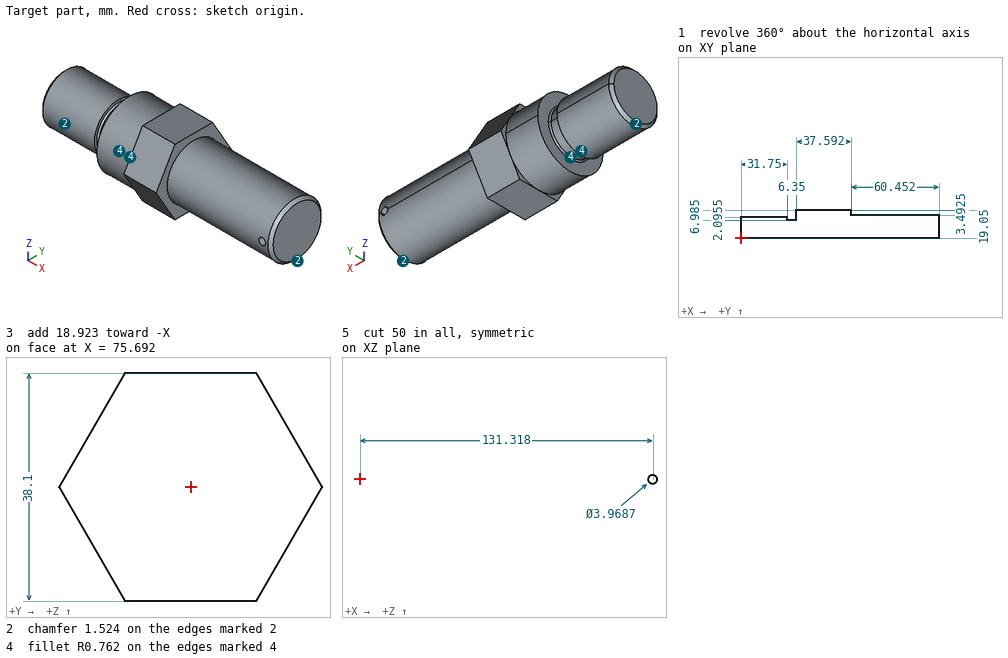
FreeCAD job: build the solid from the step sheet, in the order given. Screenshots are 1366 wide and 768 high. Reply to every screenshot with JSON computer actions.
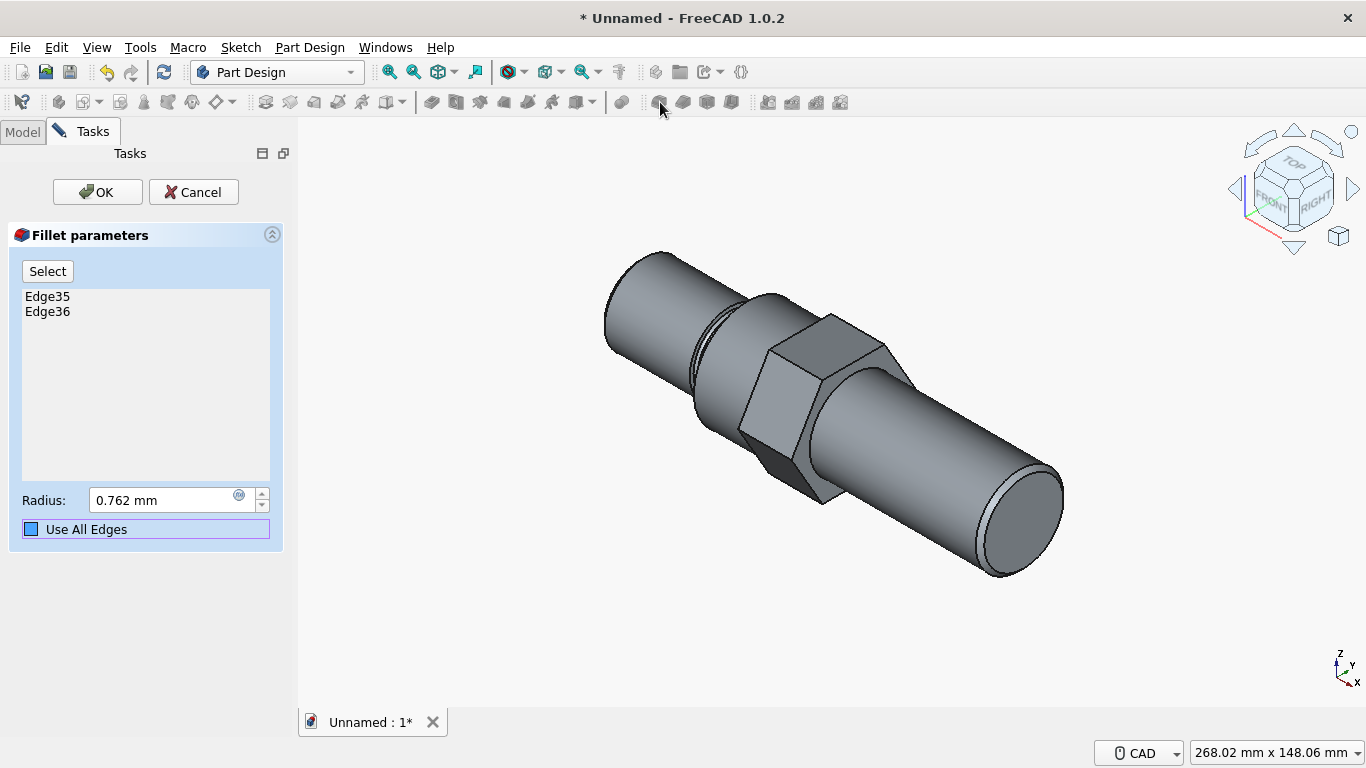
{"action": "left_click", "coordinate": [98, 192]}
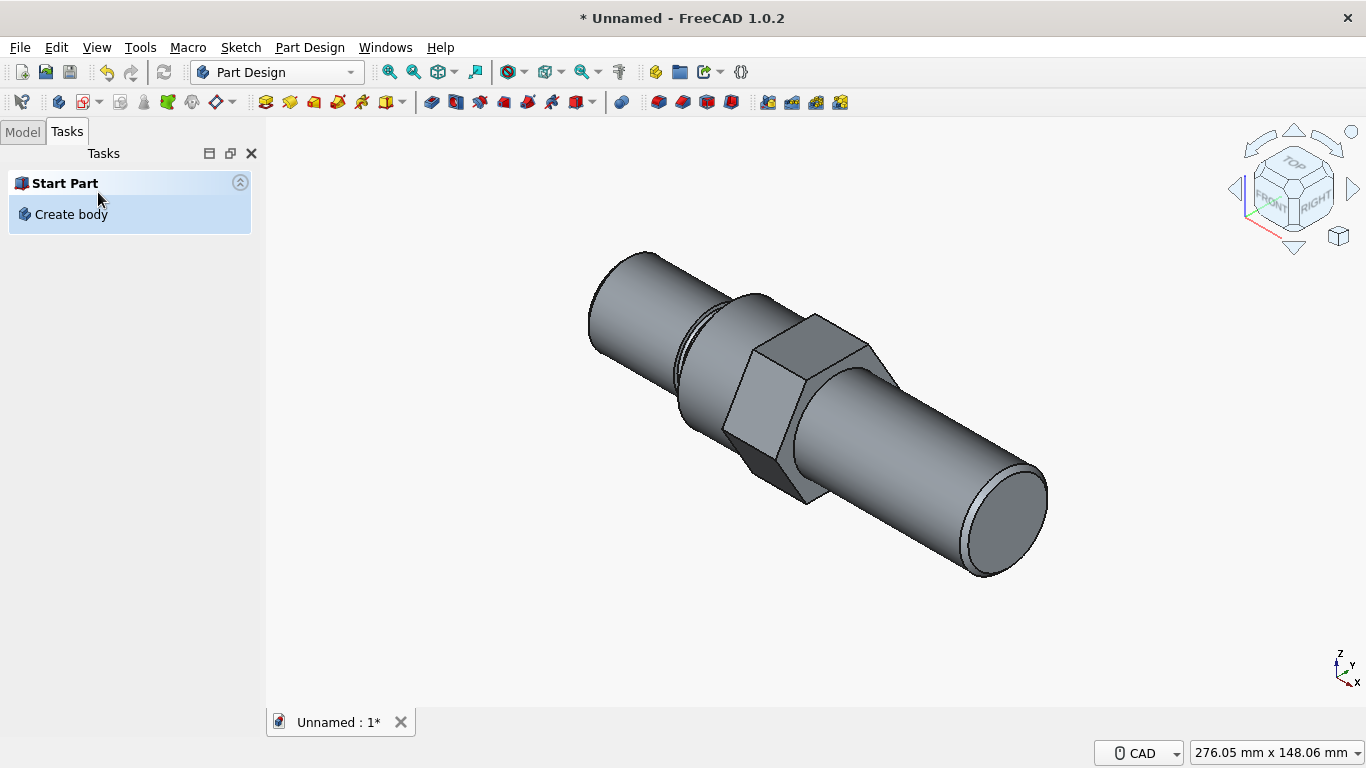
{"action": "left_click", "coordinate": [84, 102]}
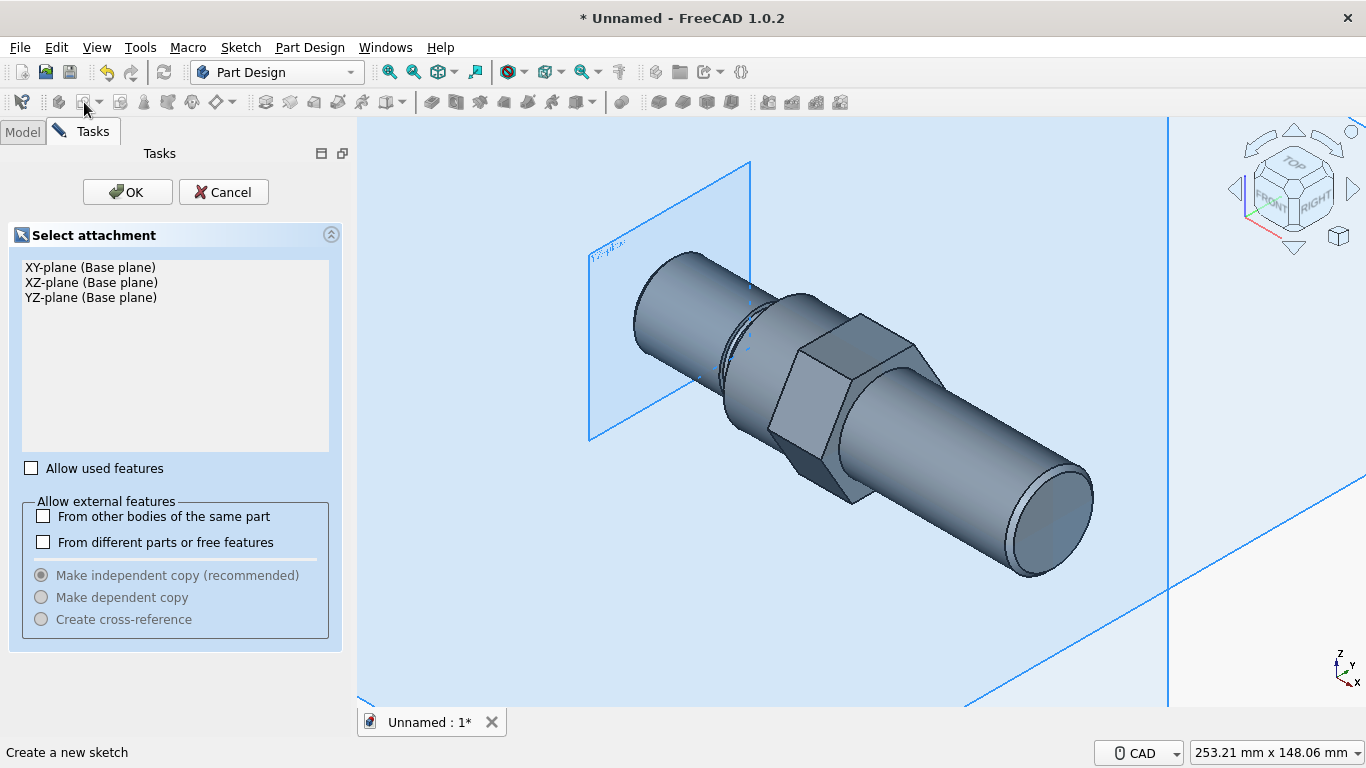
{"action": "left_click", "coordinate": [82, 282]}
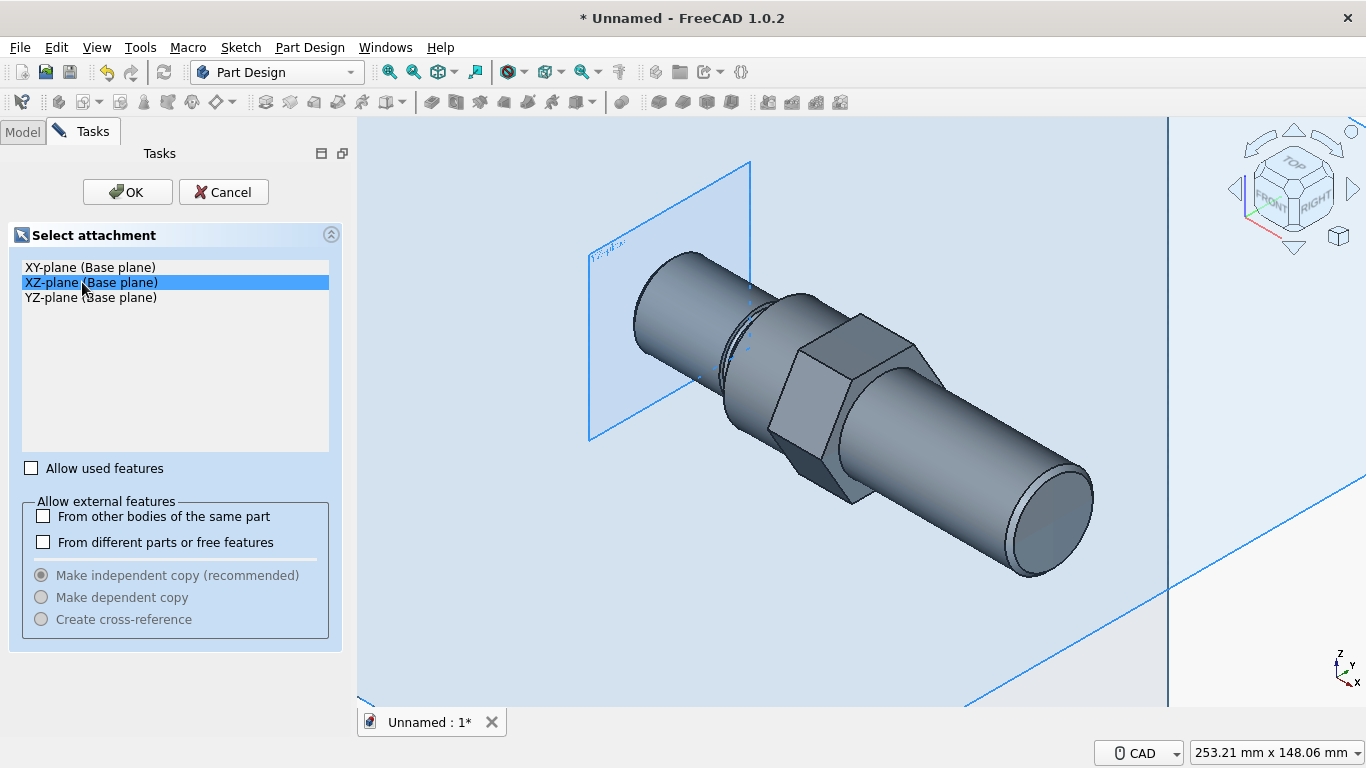
{"action": "left_click", "coordinate": [128, 192]}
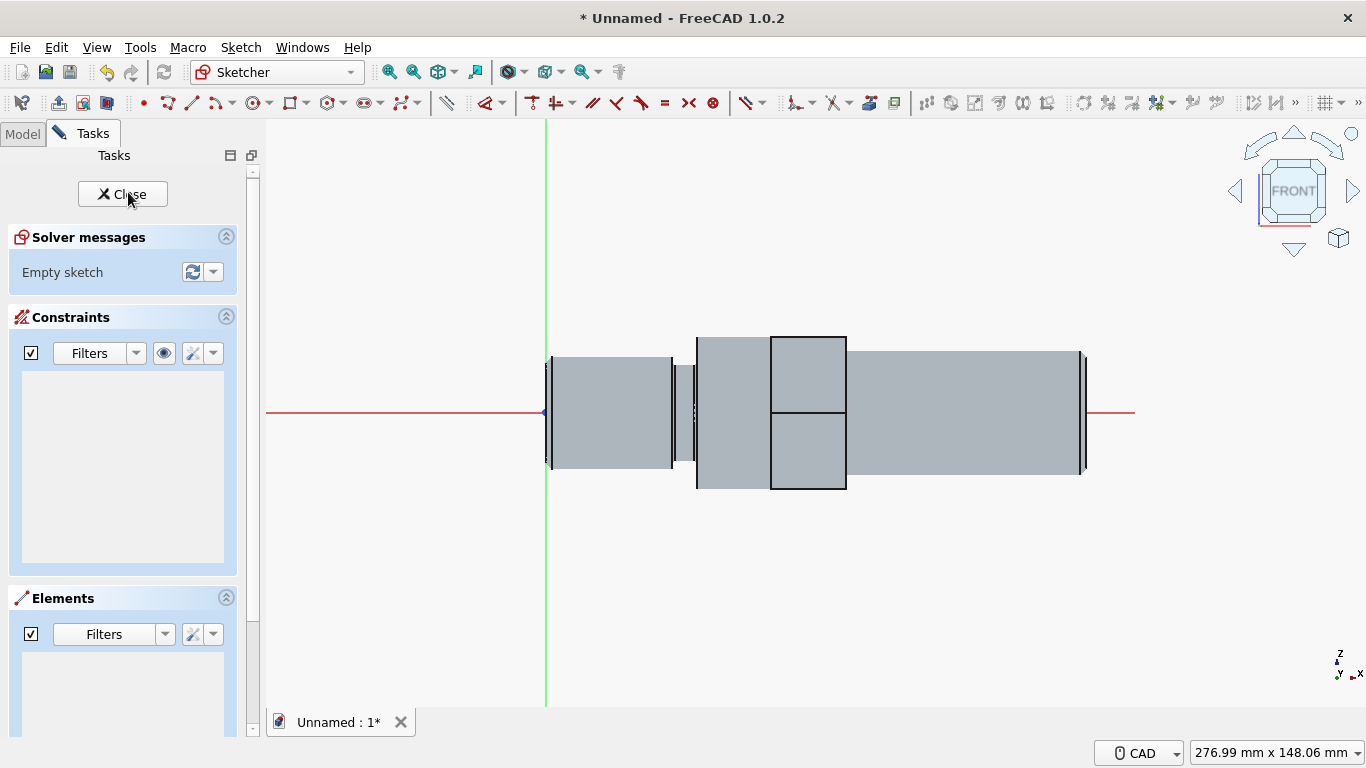
{"action": "key", "text": "q s"}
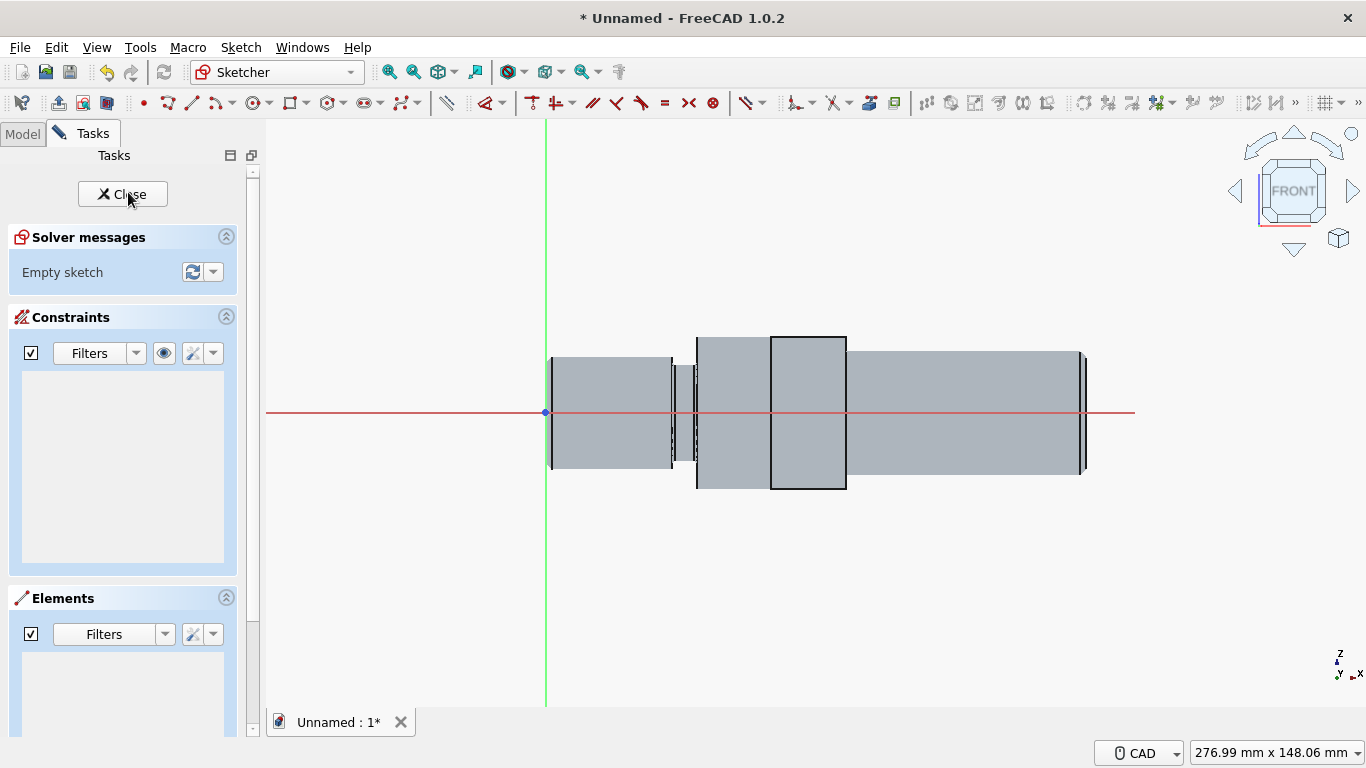
{"action": "scroll", "coordinate": [1084, 413], "scroll_direction": "up", "scroll_amount": 15}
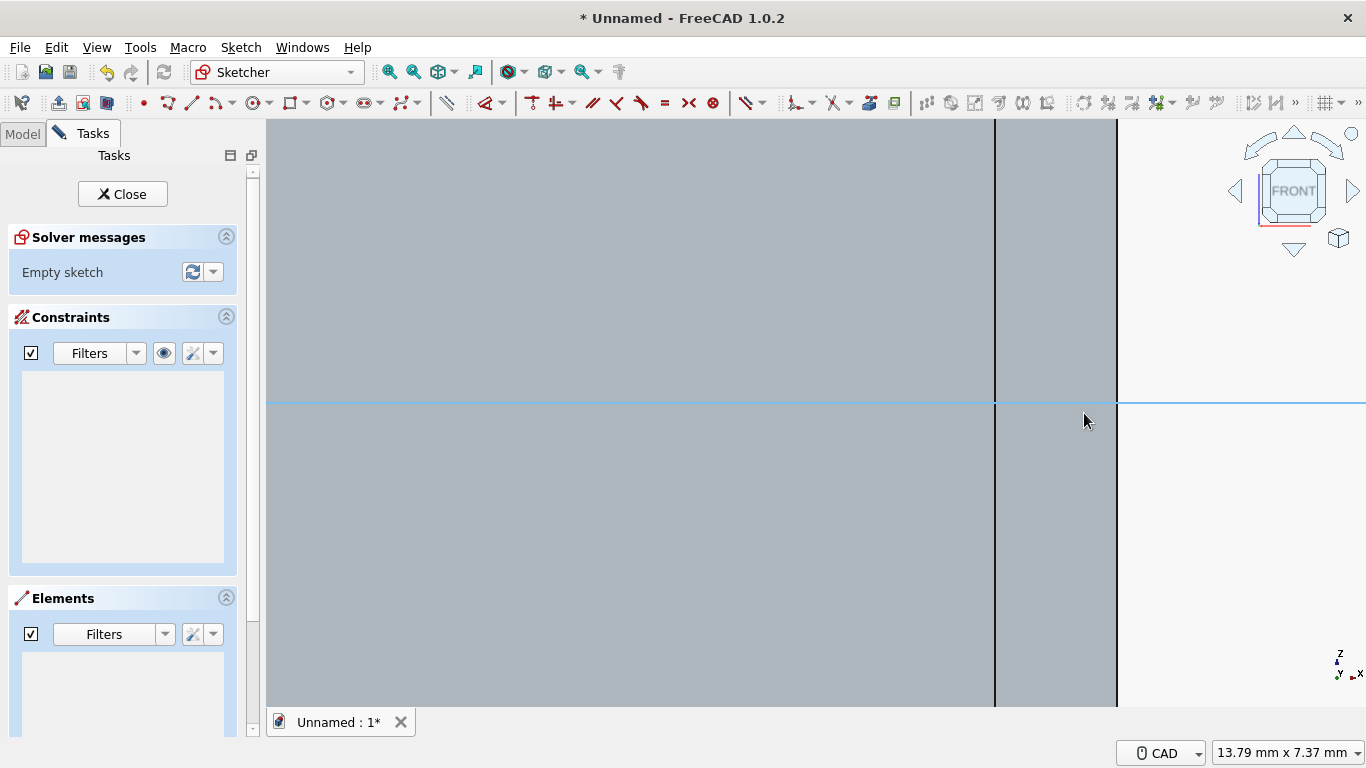
{"action": "key", "text": "g c"}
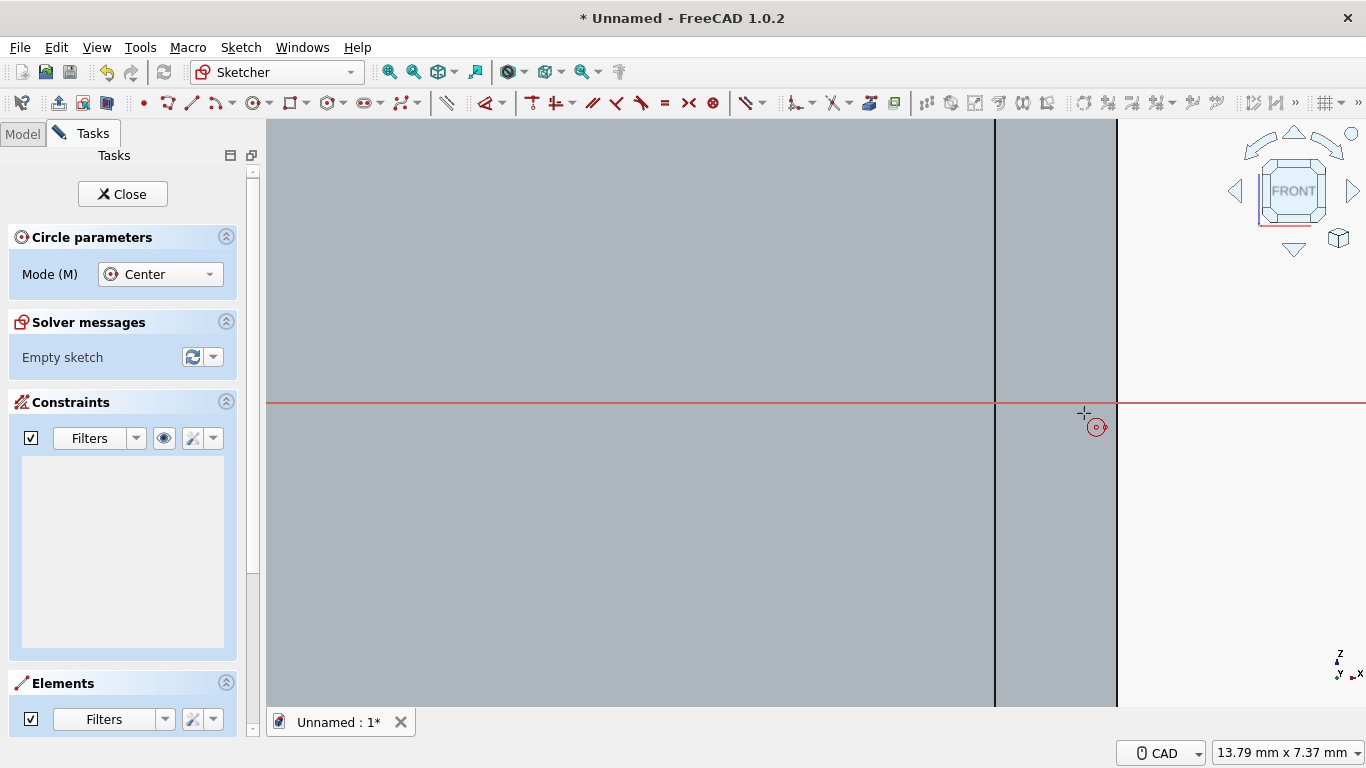
{"action": "left_click", "coordinate": [732, 403]}
{"action": "mouse_move", "coordinate": [844, 292]}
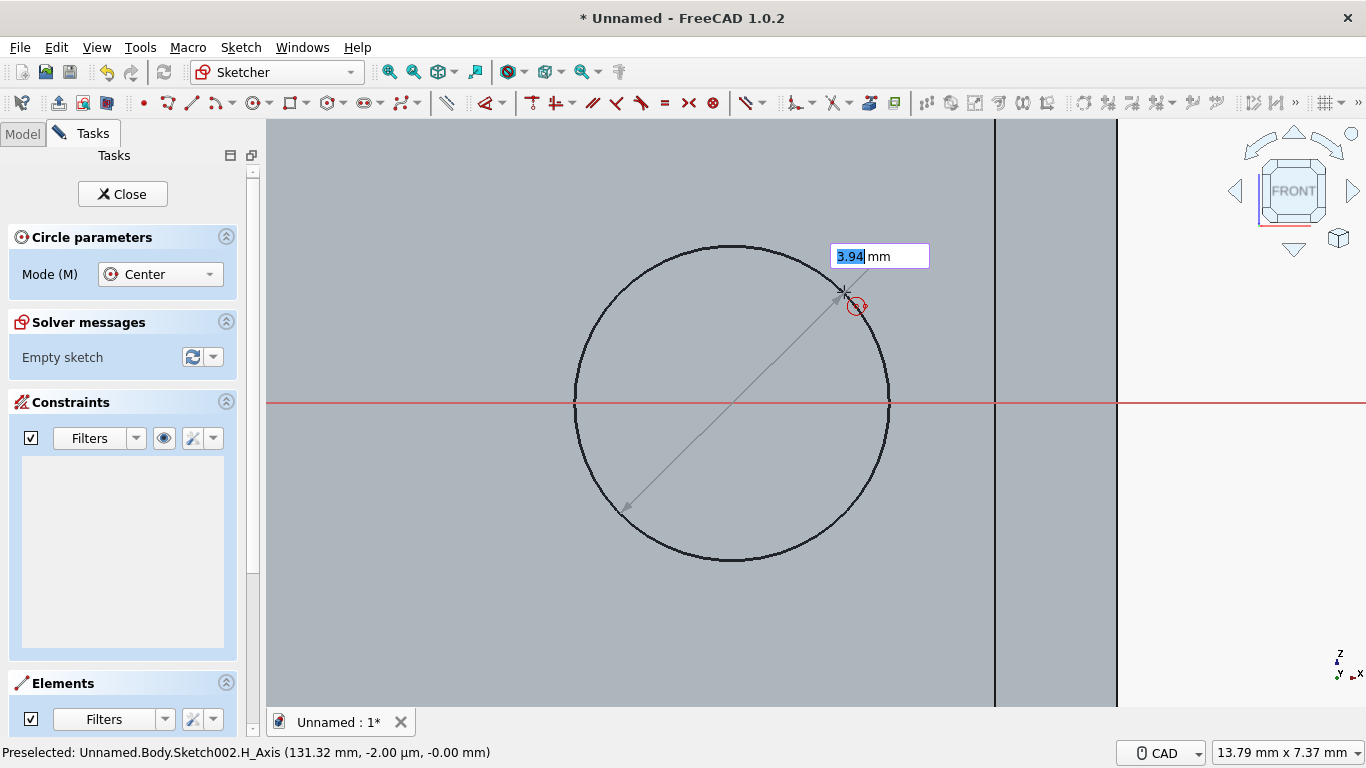
{"action": "type", "text": "3.9687"}
{"action": "key", "text": "Return"}
{"action": "key", "text": "Escape"}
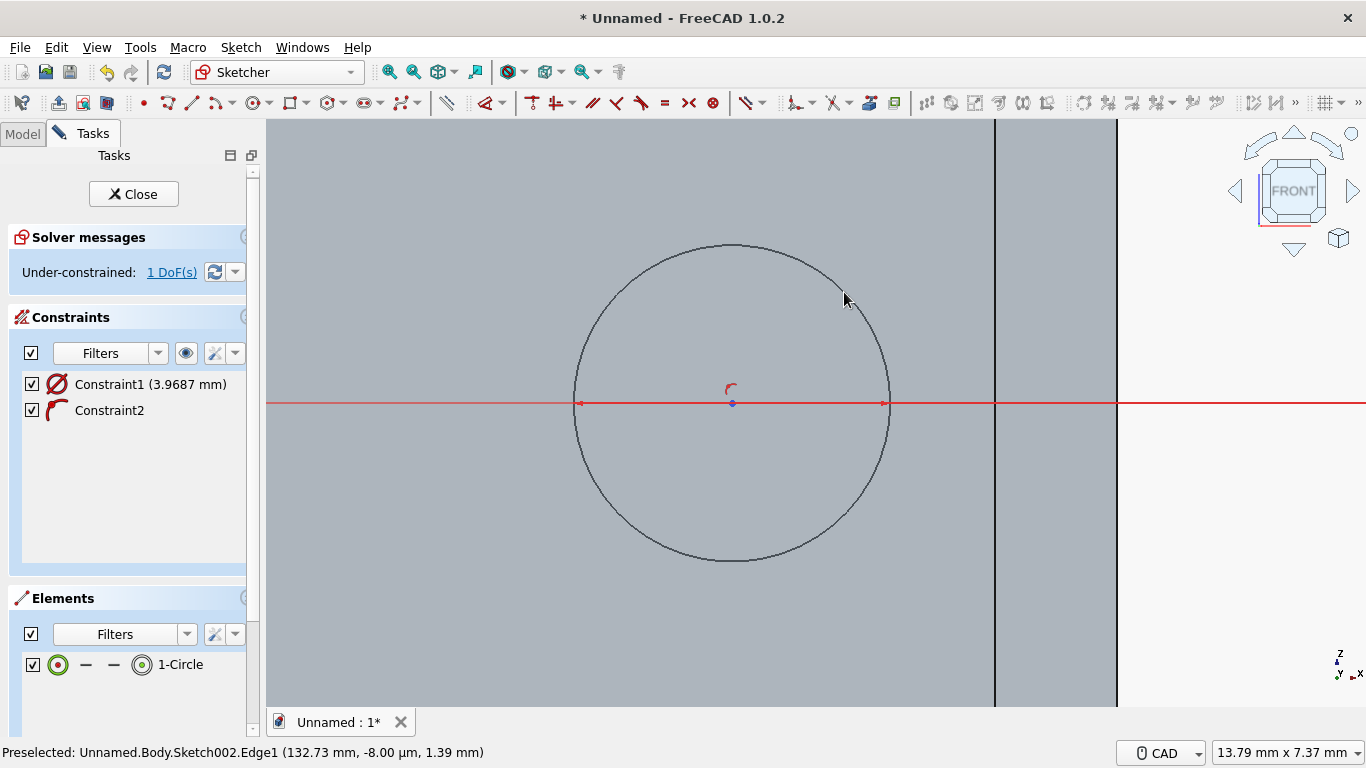
{"action": "left_click", "coordinate": [486, 104]}